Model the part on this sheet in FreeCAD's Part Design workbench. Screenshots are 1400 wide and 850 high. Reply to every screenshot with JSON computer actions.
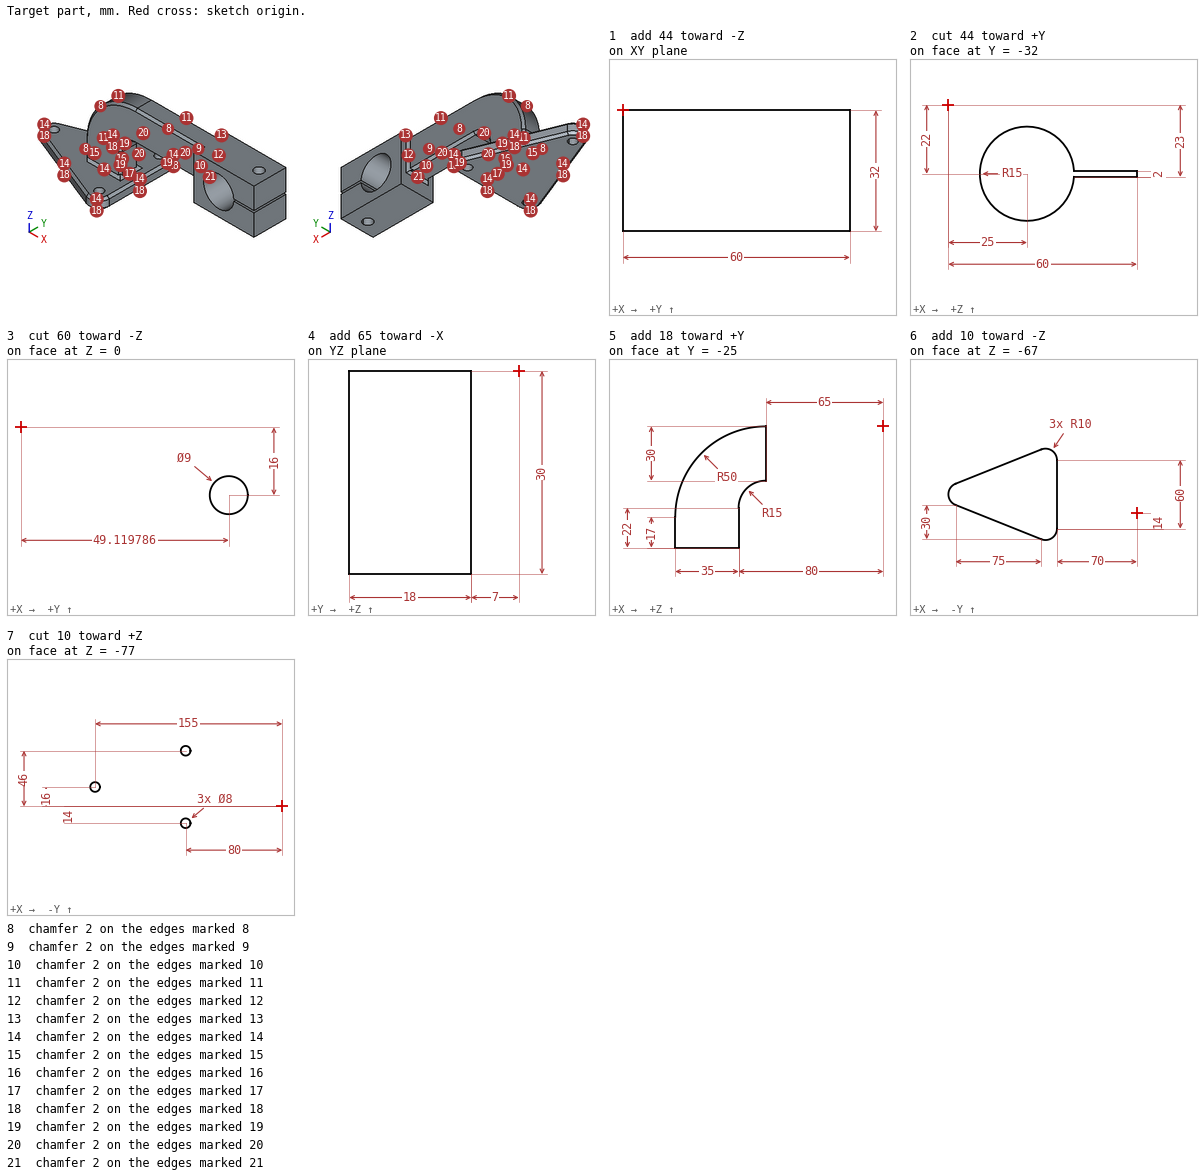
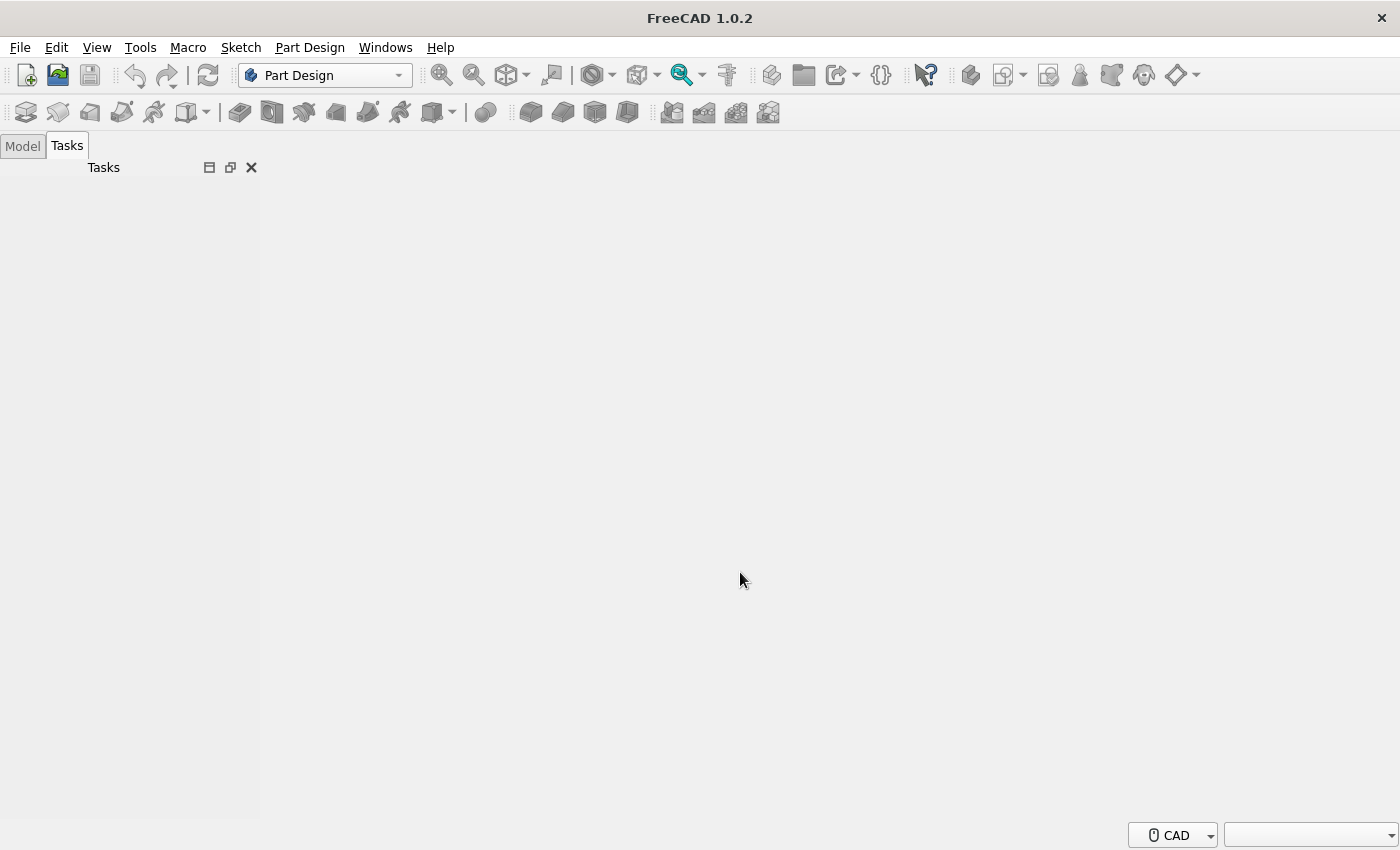
{"action": "key", "text": "ctrl+n"}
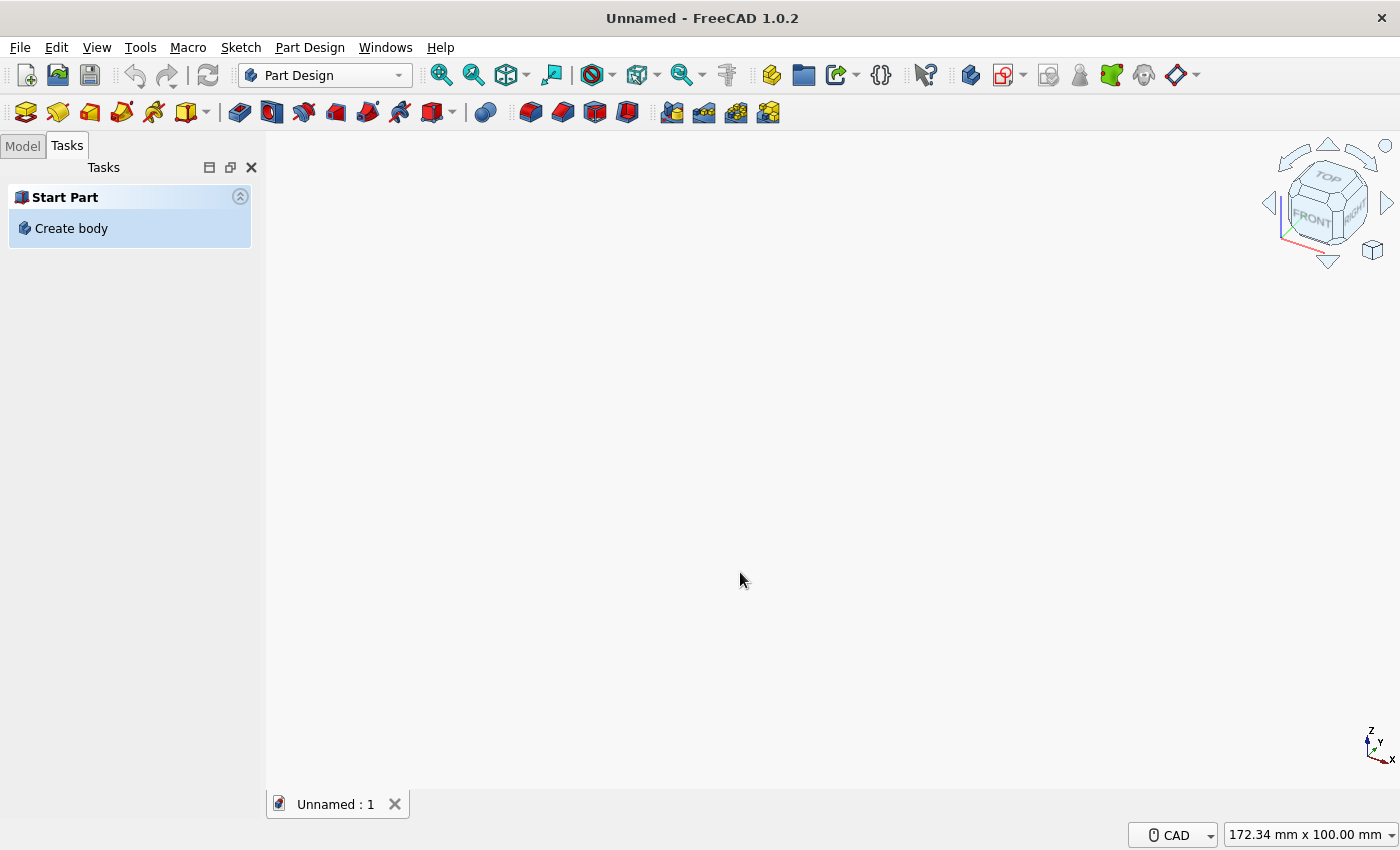
{"action": "left_click", "coordinate": [1004, 76]}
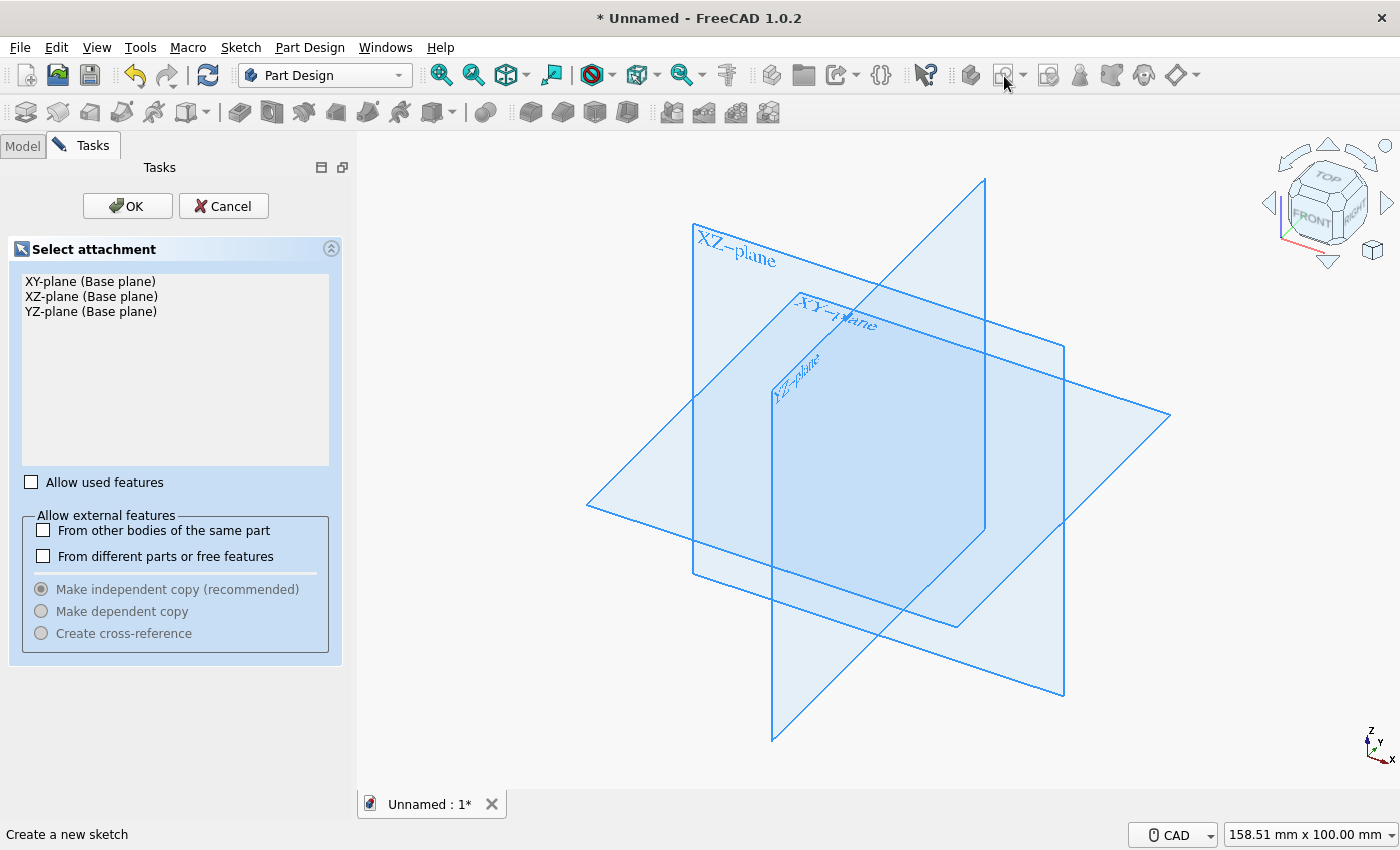
{"action": "left_click", "coordinate": [82, 282]}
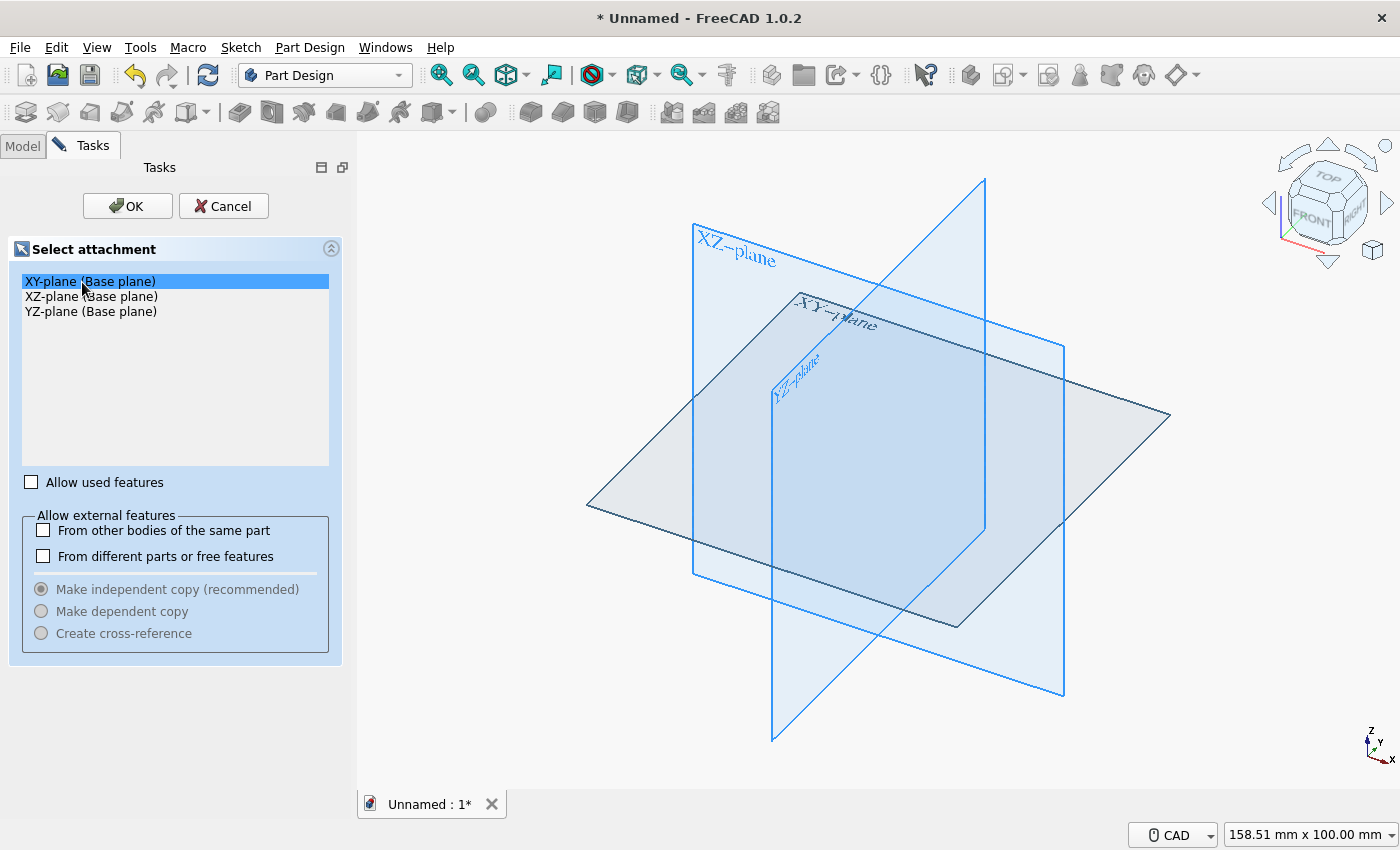
{"action": "left_click", "coordinate": [128, 206]}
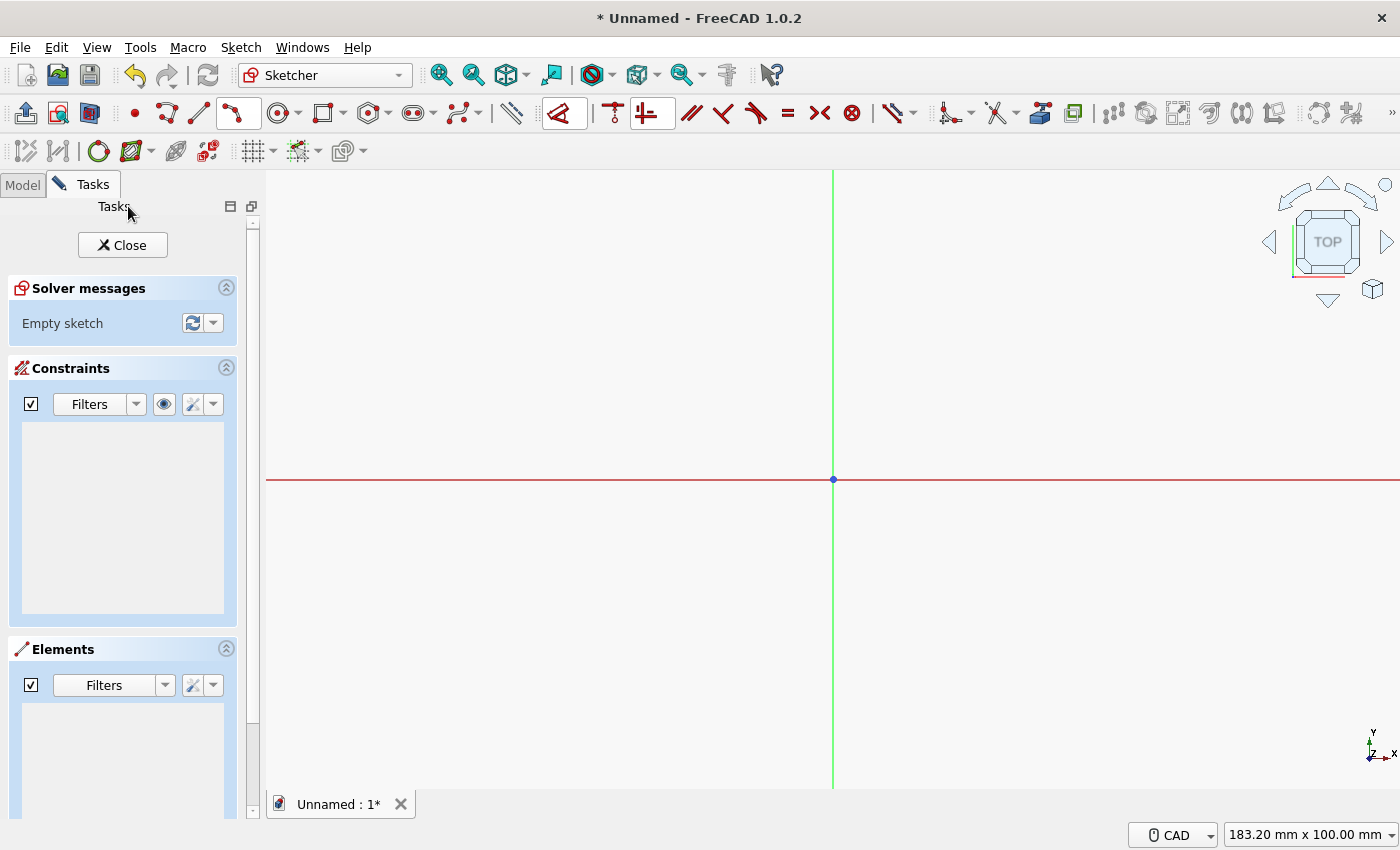
{"action": "scroll", "coordinate": [1235, 699], "scroll_direction": "up", "scroll_amount": 3}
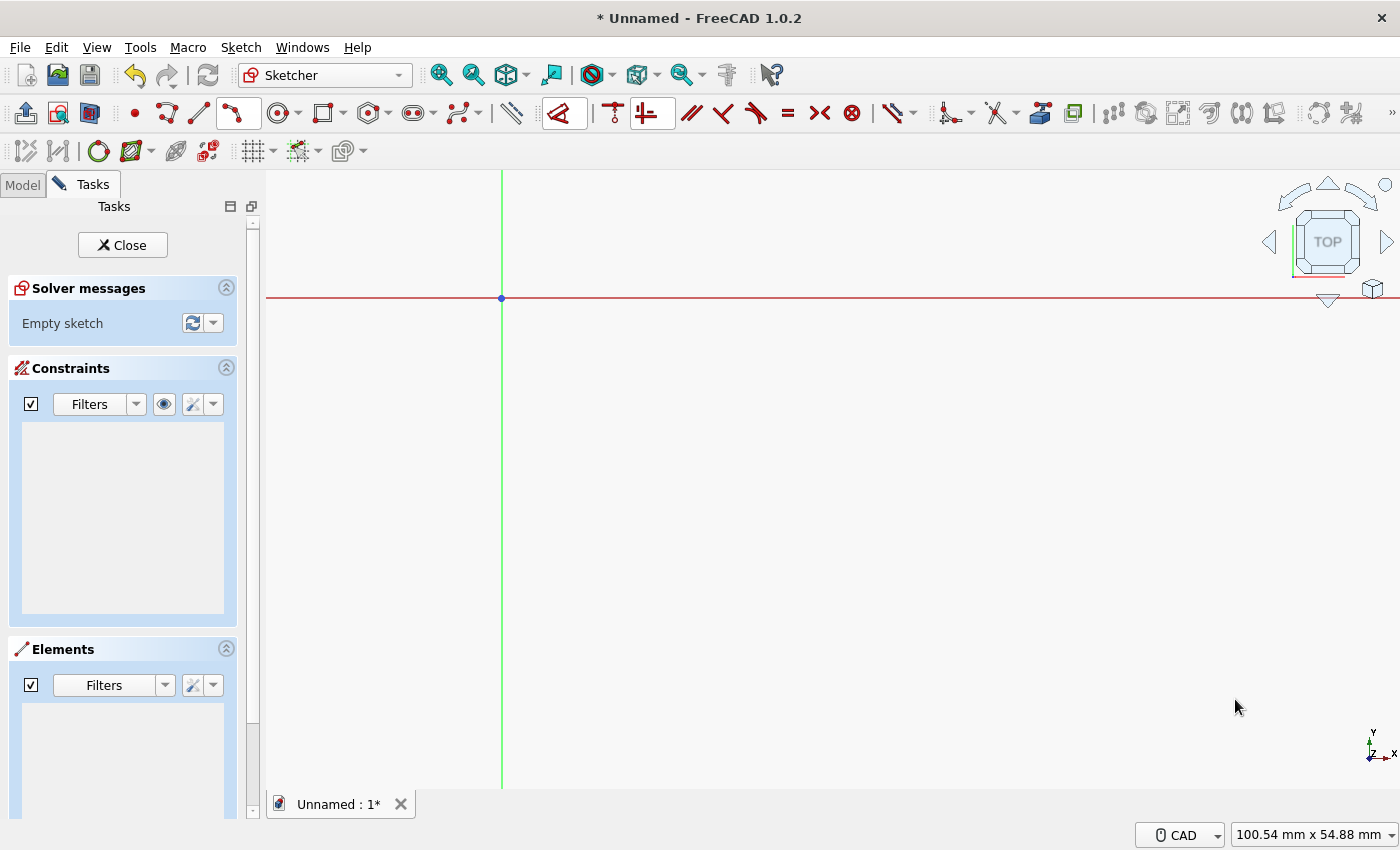
{"action": "left_click", "coordinate": [324, 114]}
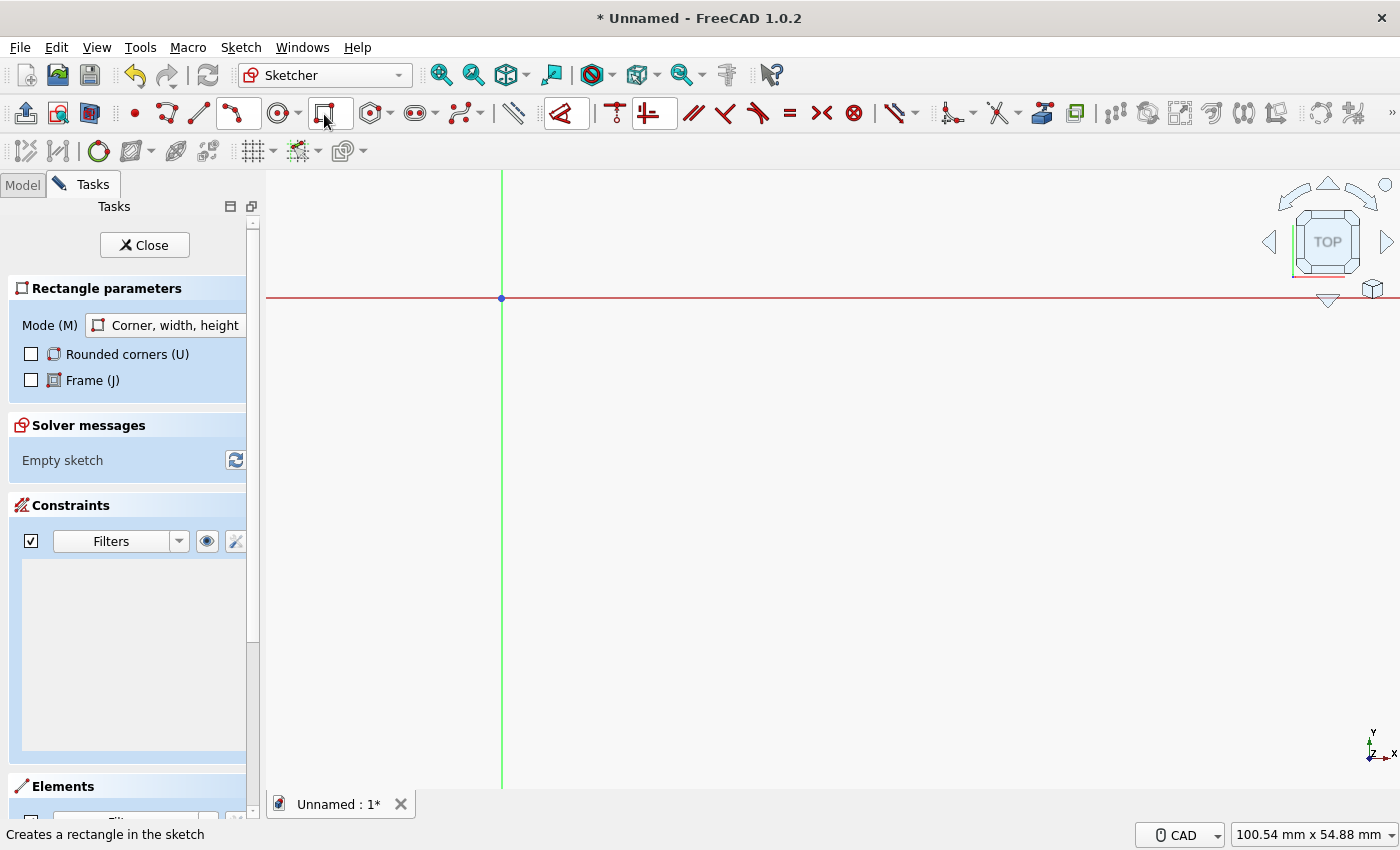
{"action": "left_click", "coordinate": [502, 298]}
{"action": "mouse_move", "coordinate": [1179, 659]}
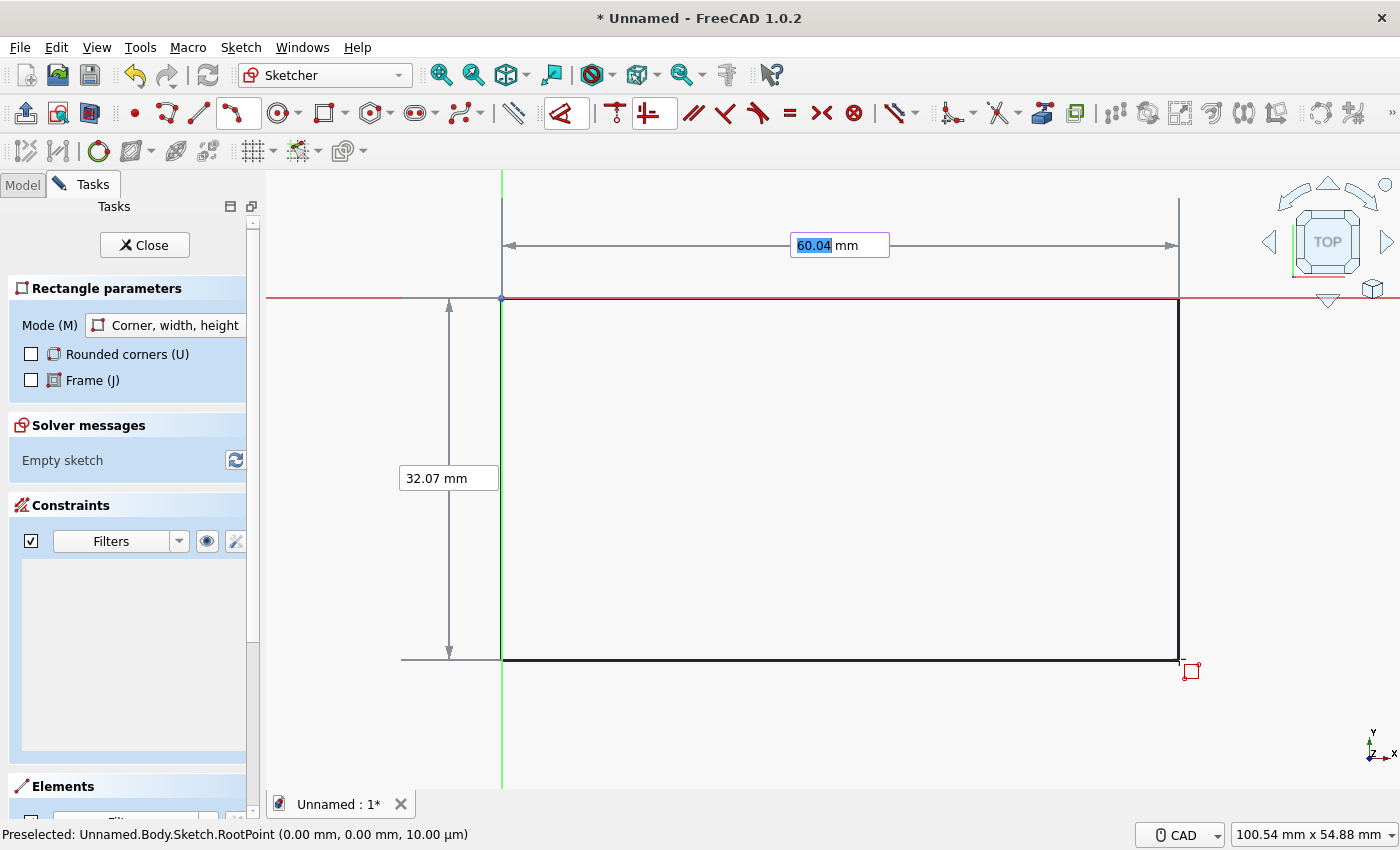
{"action": "type", "text": "60"}
{"action": "key", "text": "Tab"}
{"action": "type", "text": "32"}
{"action": "key", "text": "Return"}
{"action": "key", "text": "Escape"}